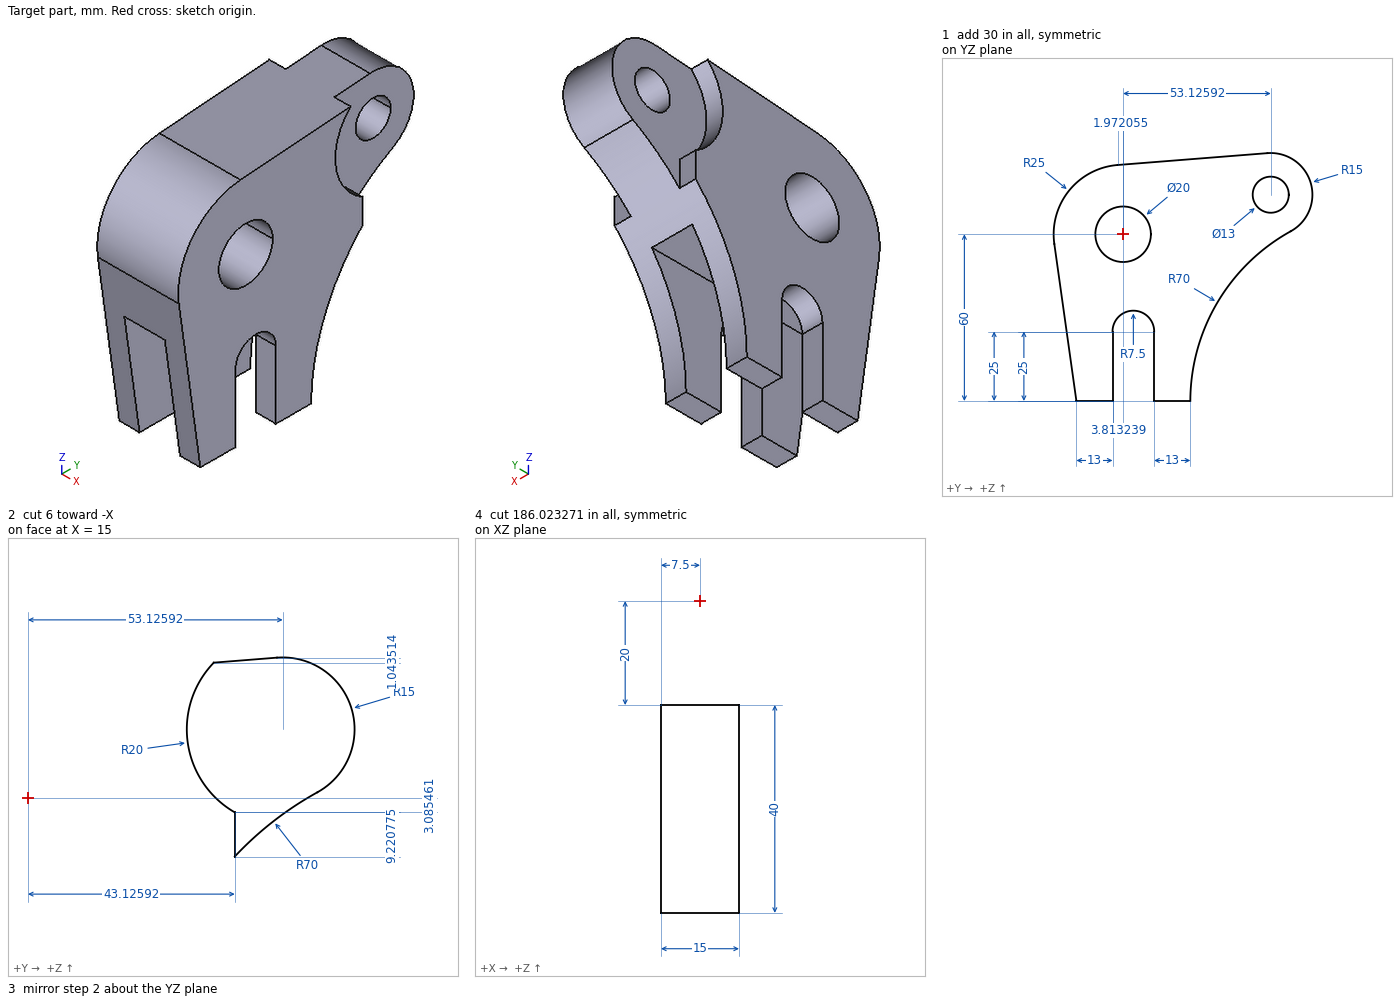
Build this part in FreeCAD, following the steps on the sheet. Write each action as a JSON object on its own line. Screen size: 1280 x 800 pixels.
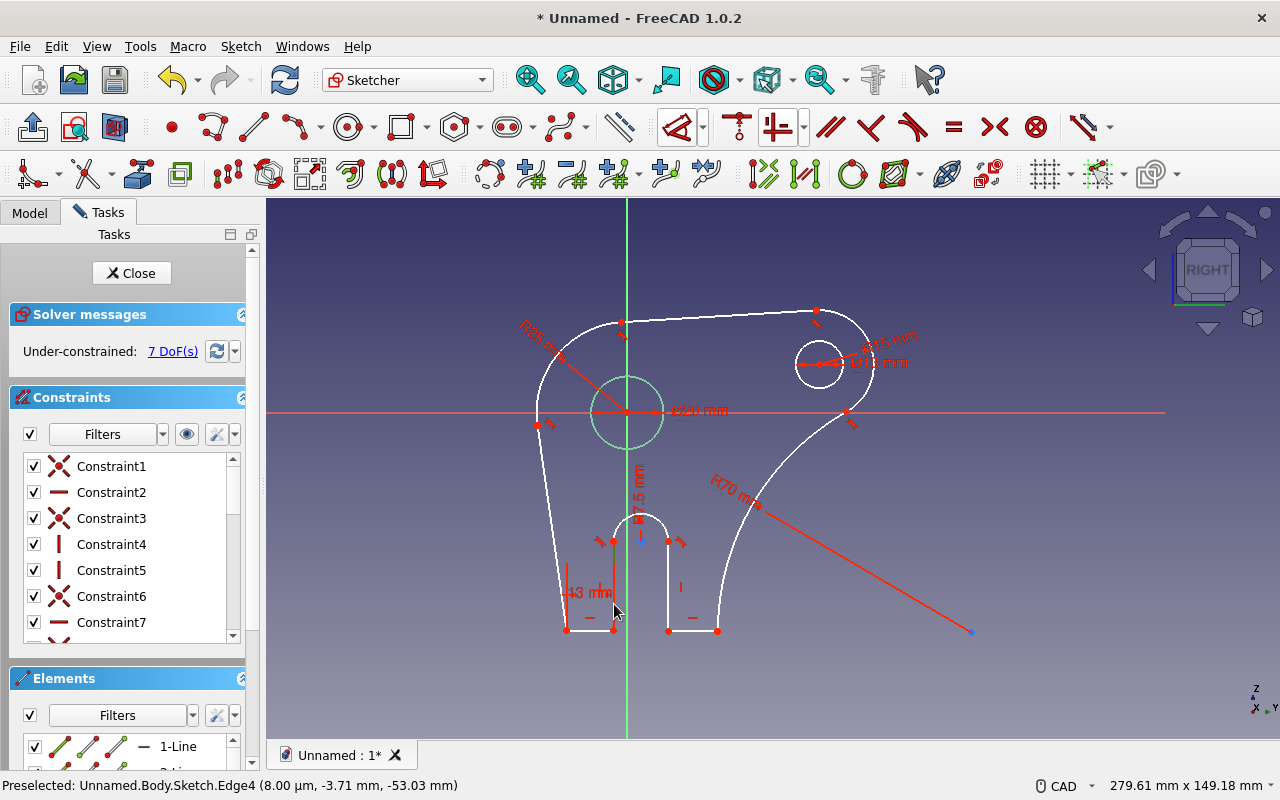
{"action": "key", "text": "i"}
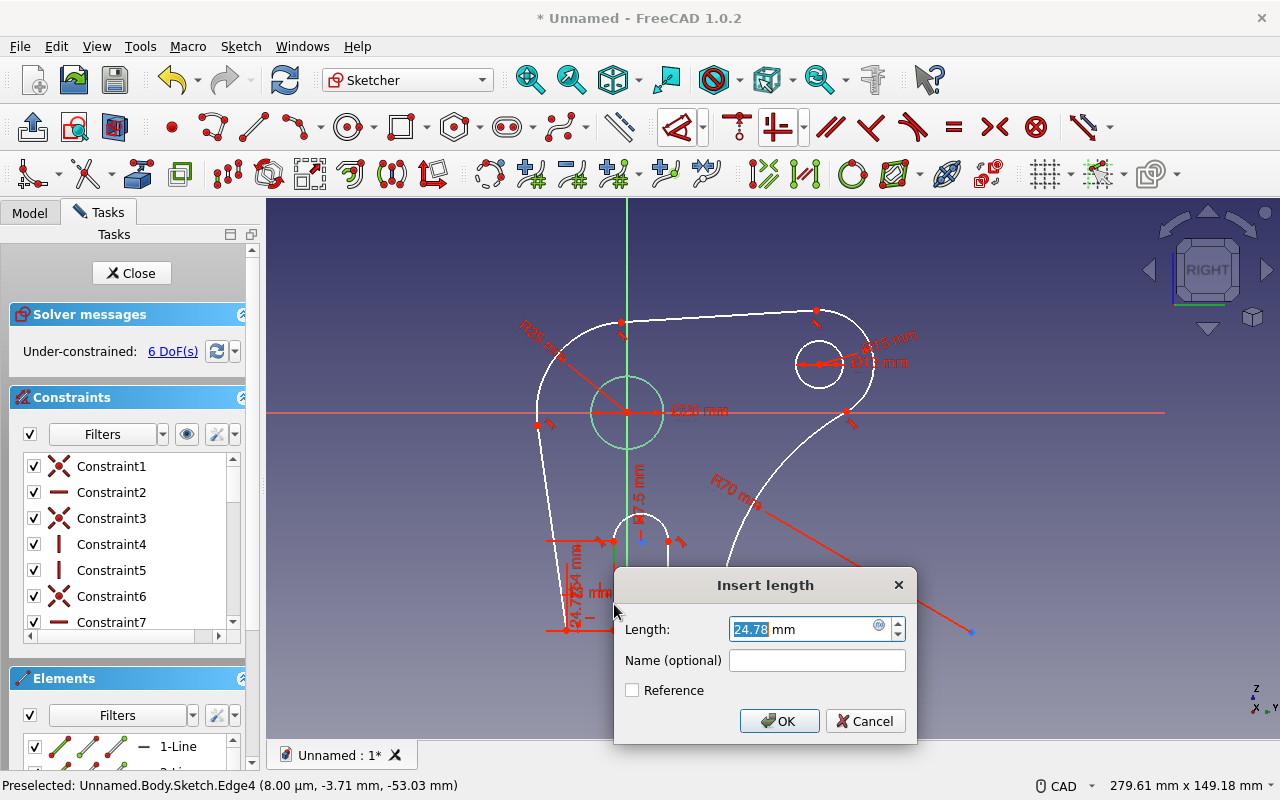
{"action": "type", "text": "25"}
{"action": "key", "text": "Return"}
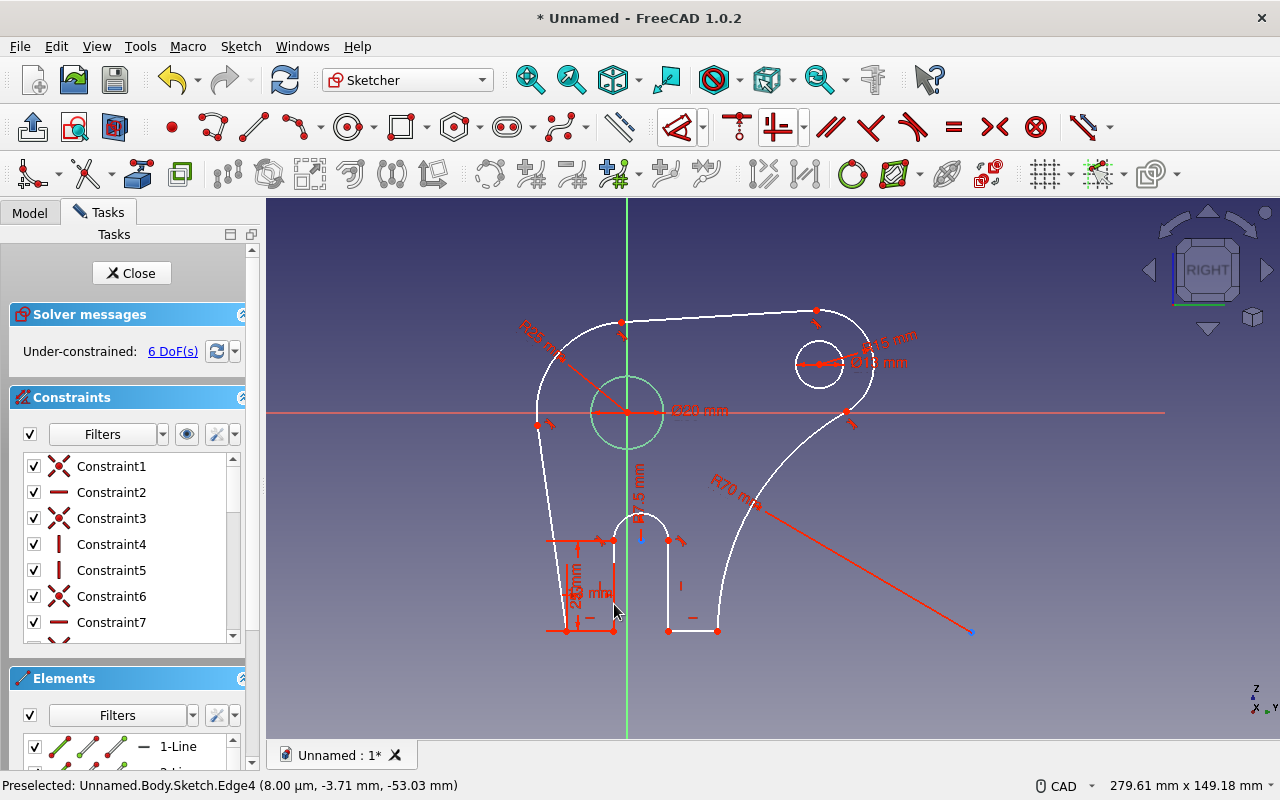
{"action": "left_click", "coordinate": [668, 568]}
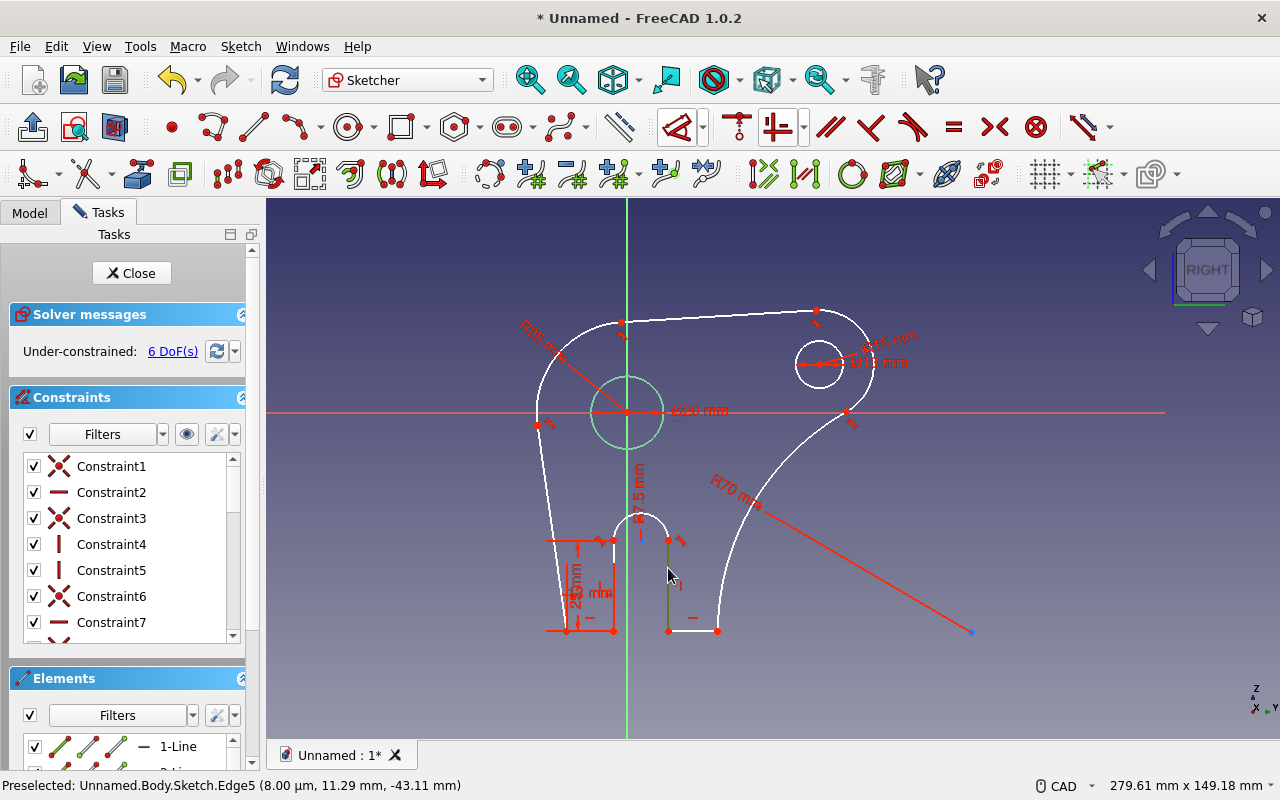
{"action": "left_click", "coordinate": [702, 128]}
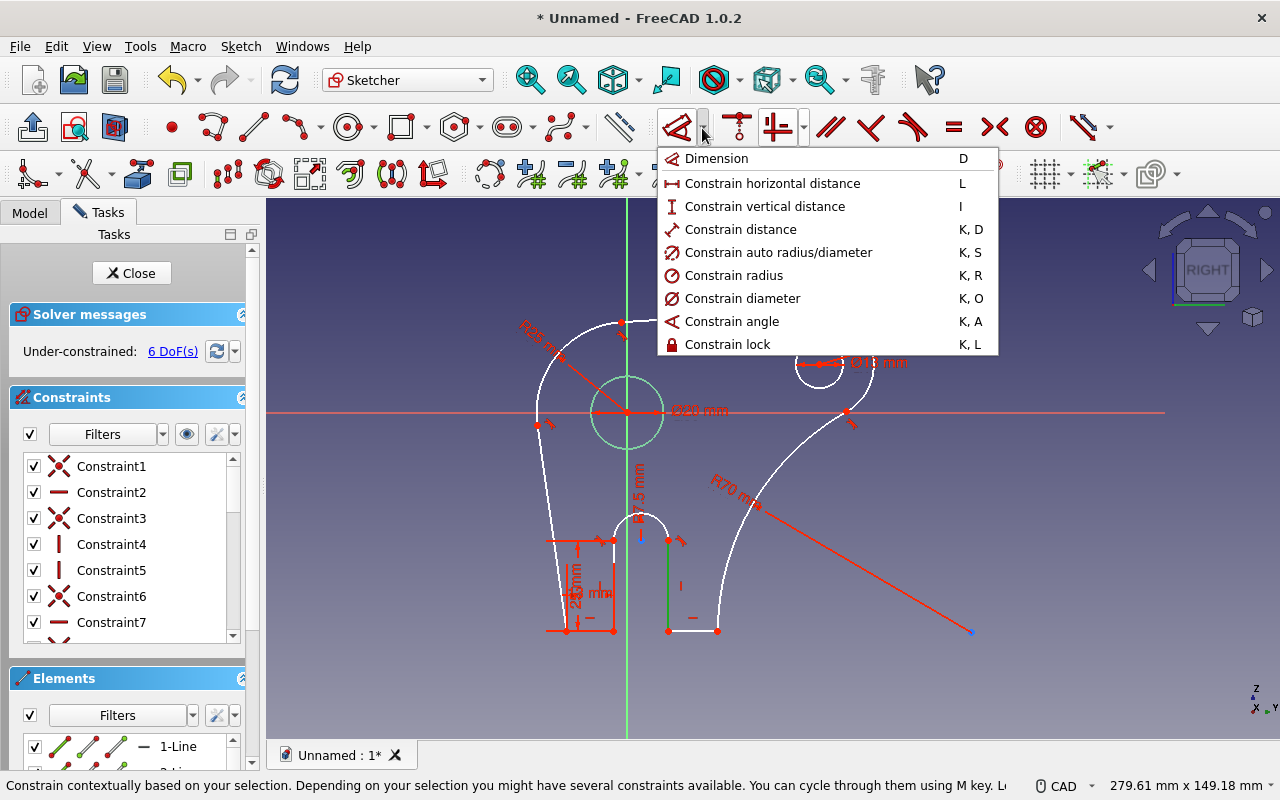
{"action": "left_click", "coordinate": [828, 206]}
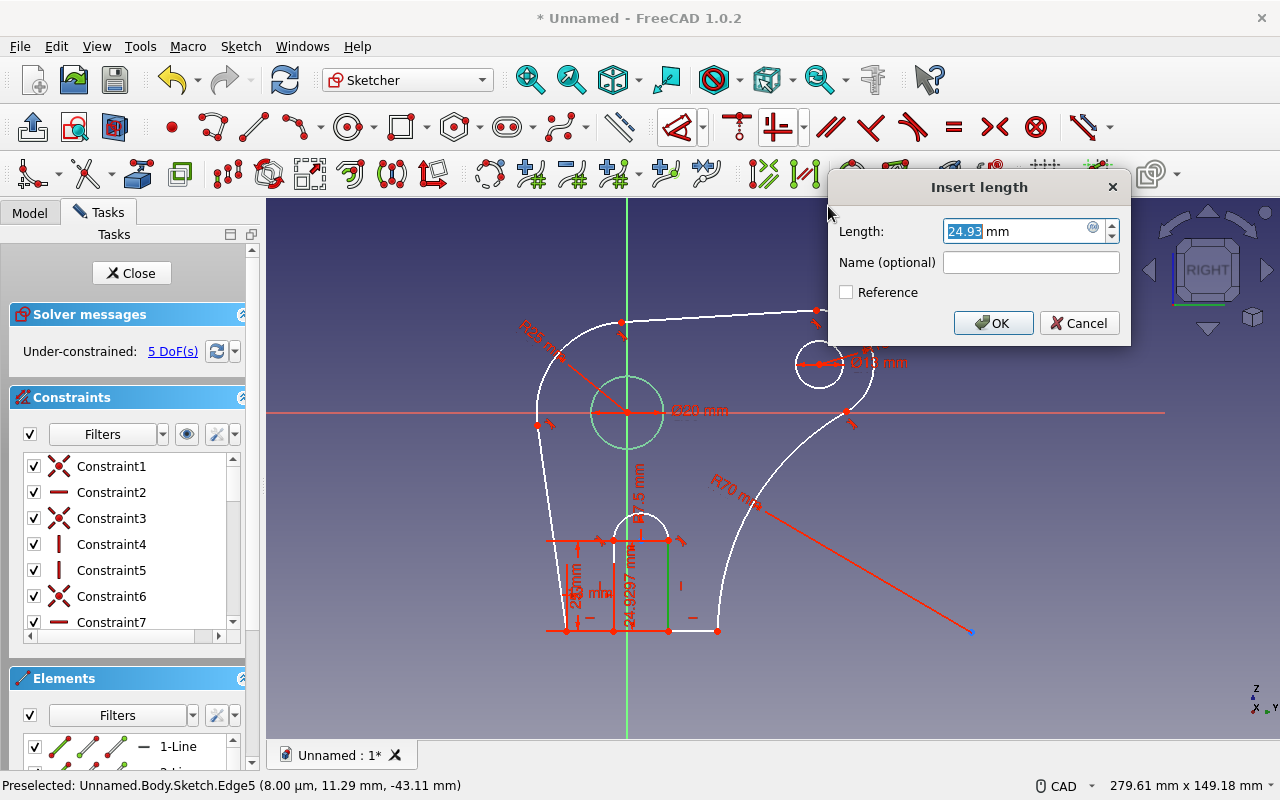
{"action": "type", "text": "25"}
{"action": "key", "text": "Return"}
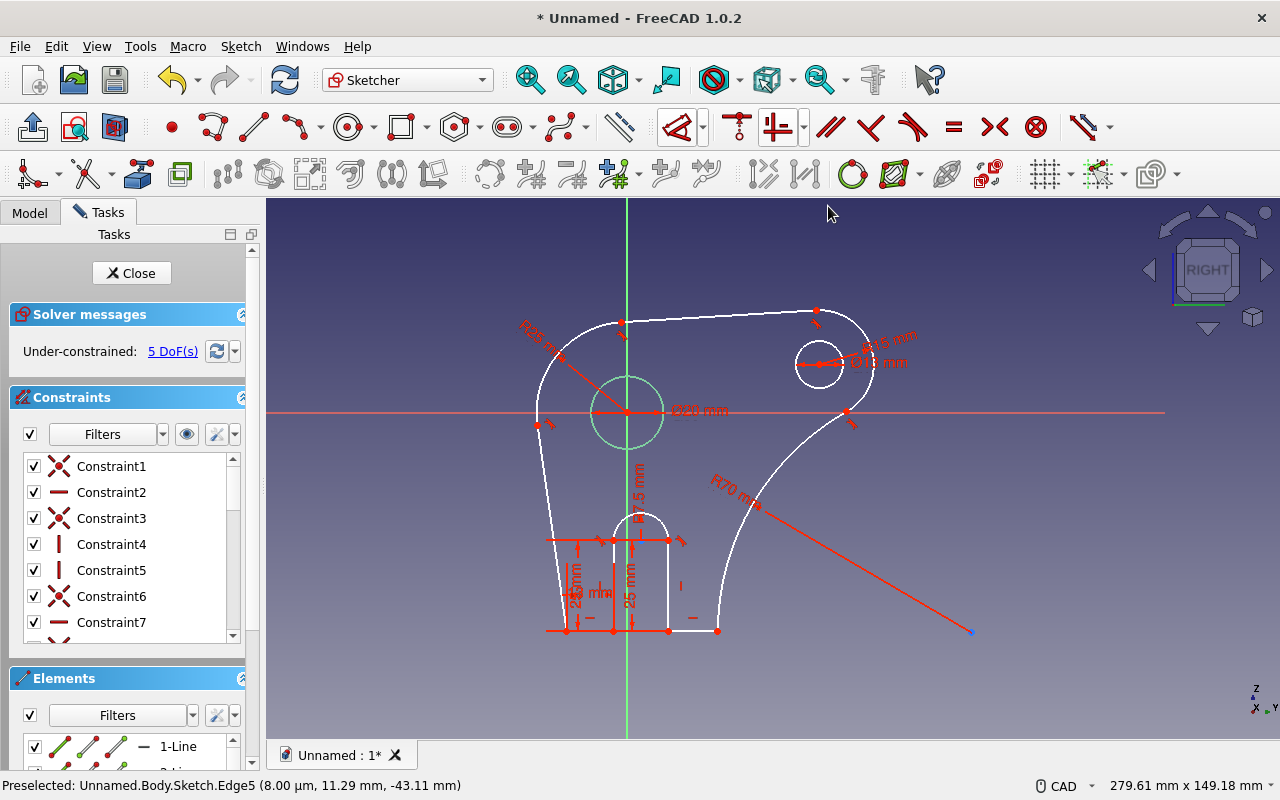
{"action": "left_click", "coordinate": [683, 631]}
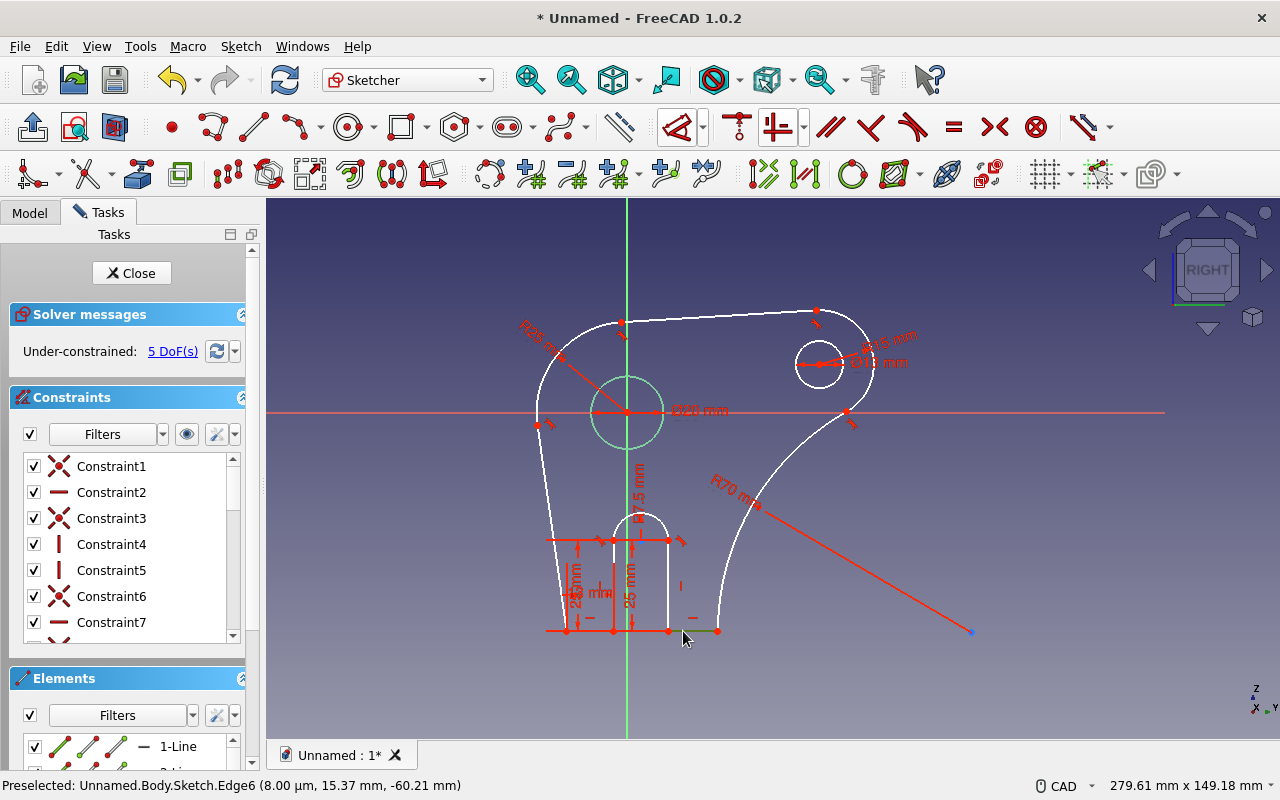
{"action": "left_click", "coordinate": [702, 128]}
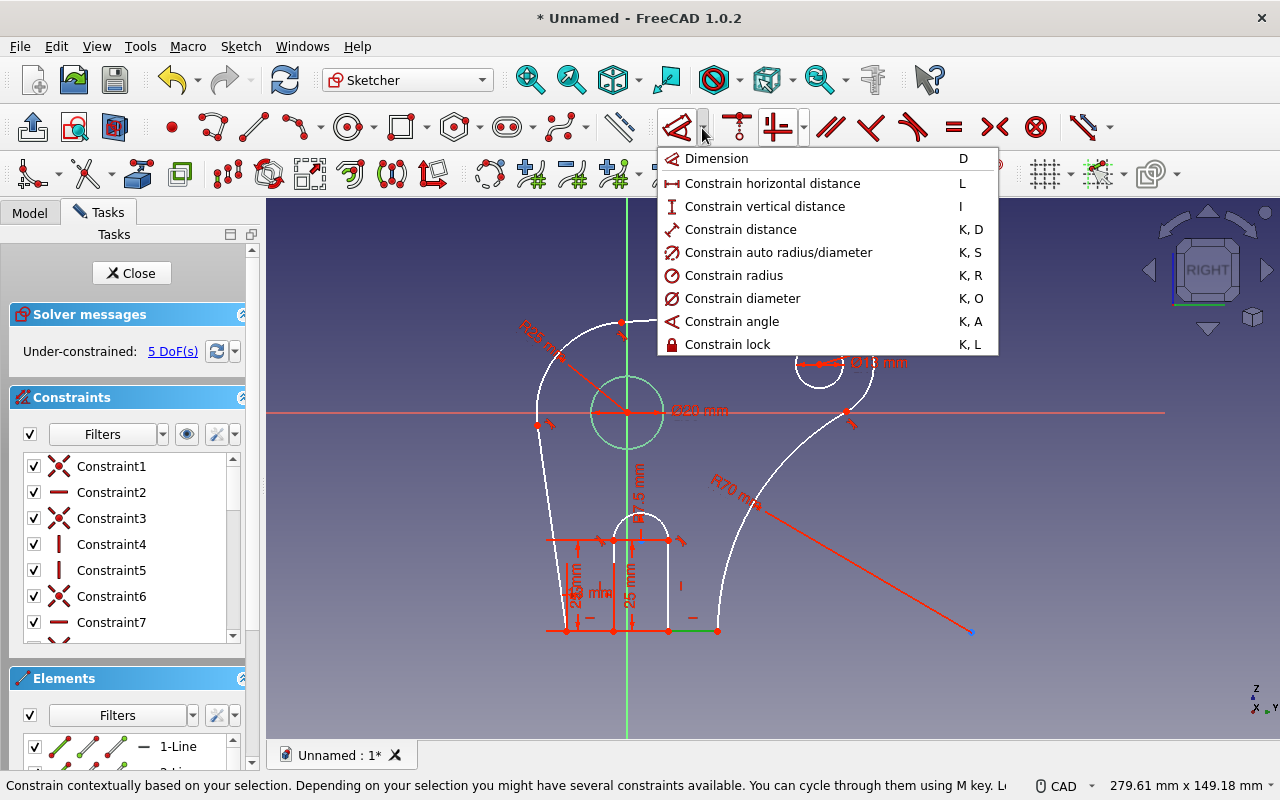
{"action": "left_click", "coordinate": [828, 184]}